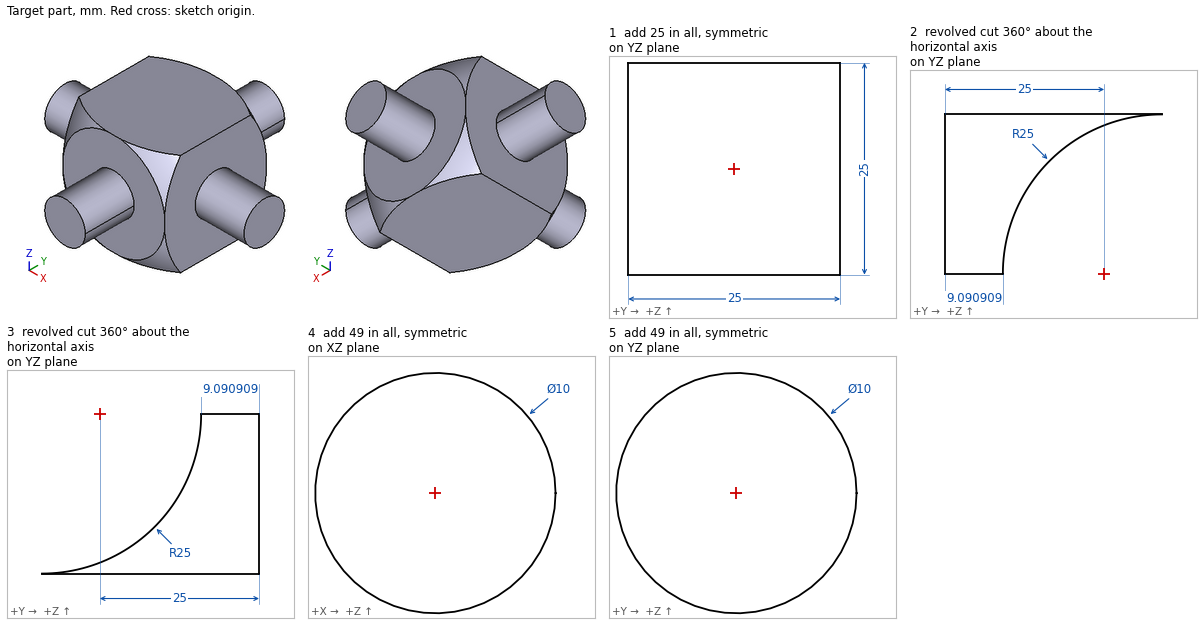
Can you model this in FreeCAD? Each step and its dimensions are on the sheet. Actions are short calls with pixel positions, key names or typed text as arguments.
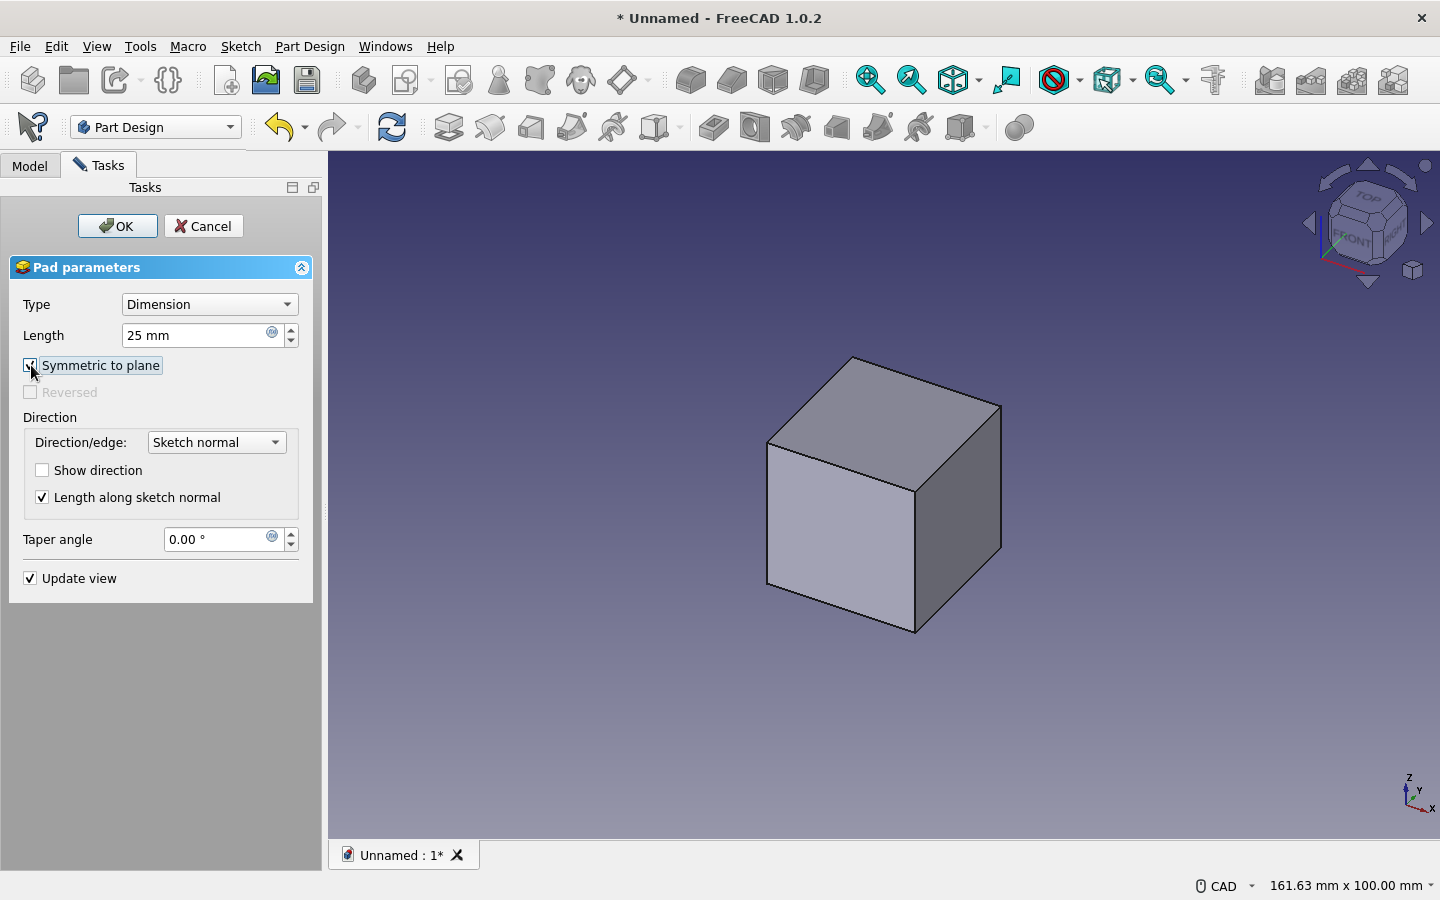
click(118, 226)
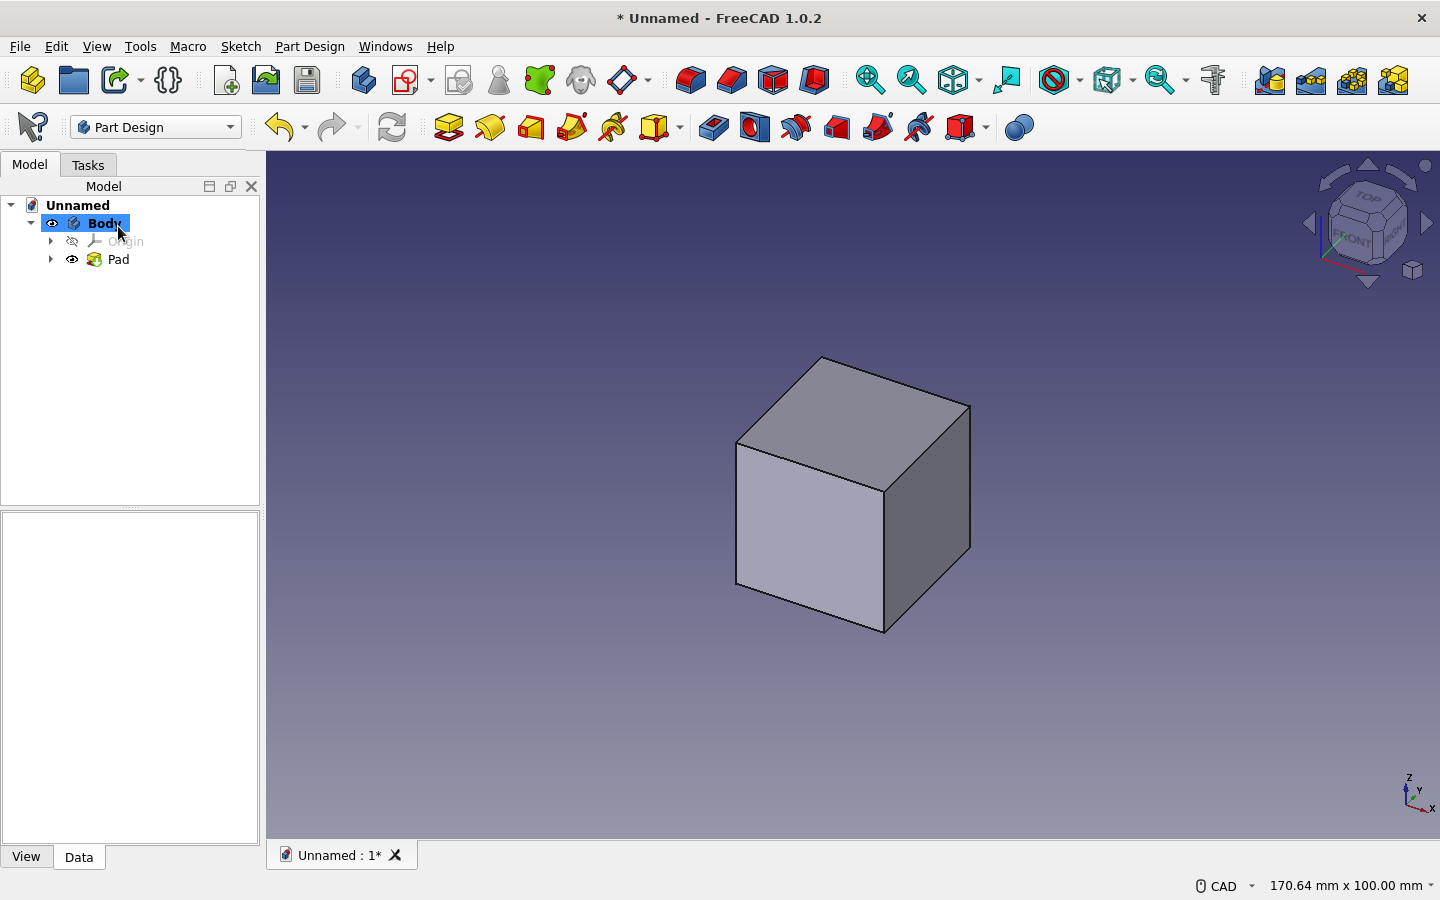
key(v)
key(f)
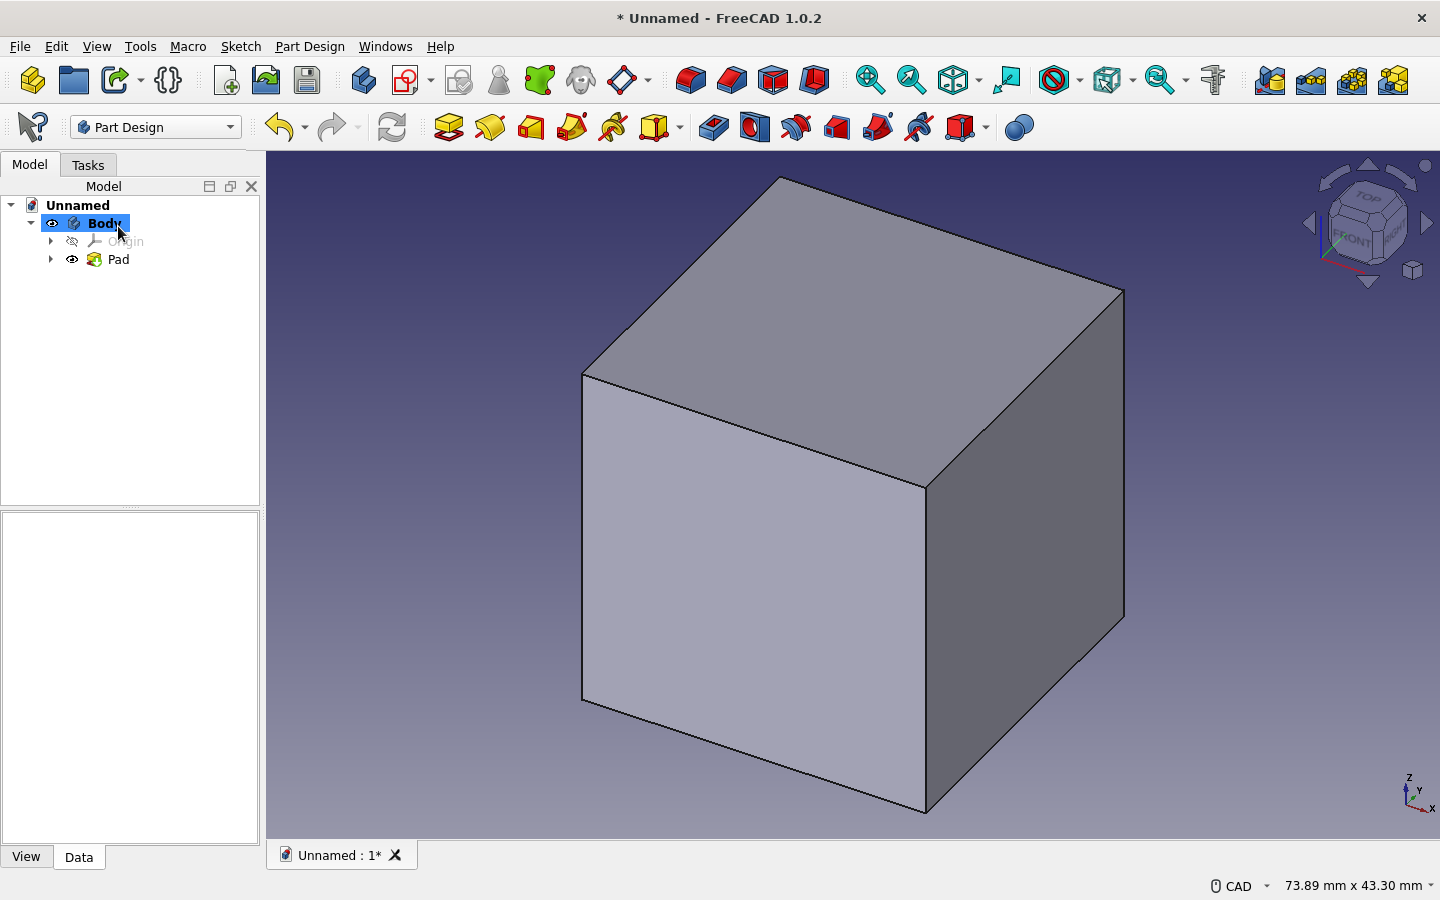
click(404, 80)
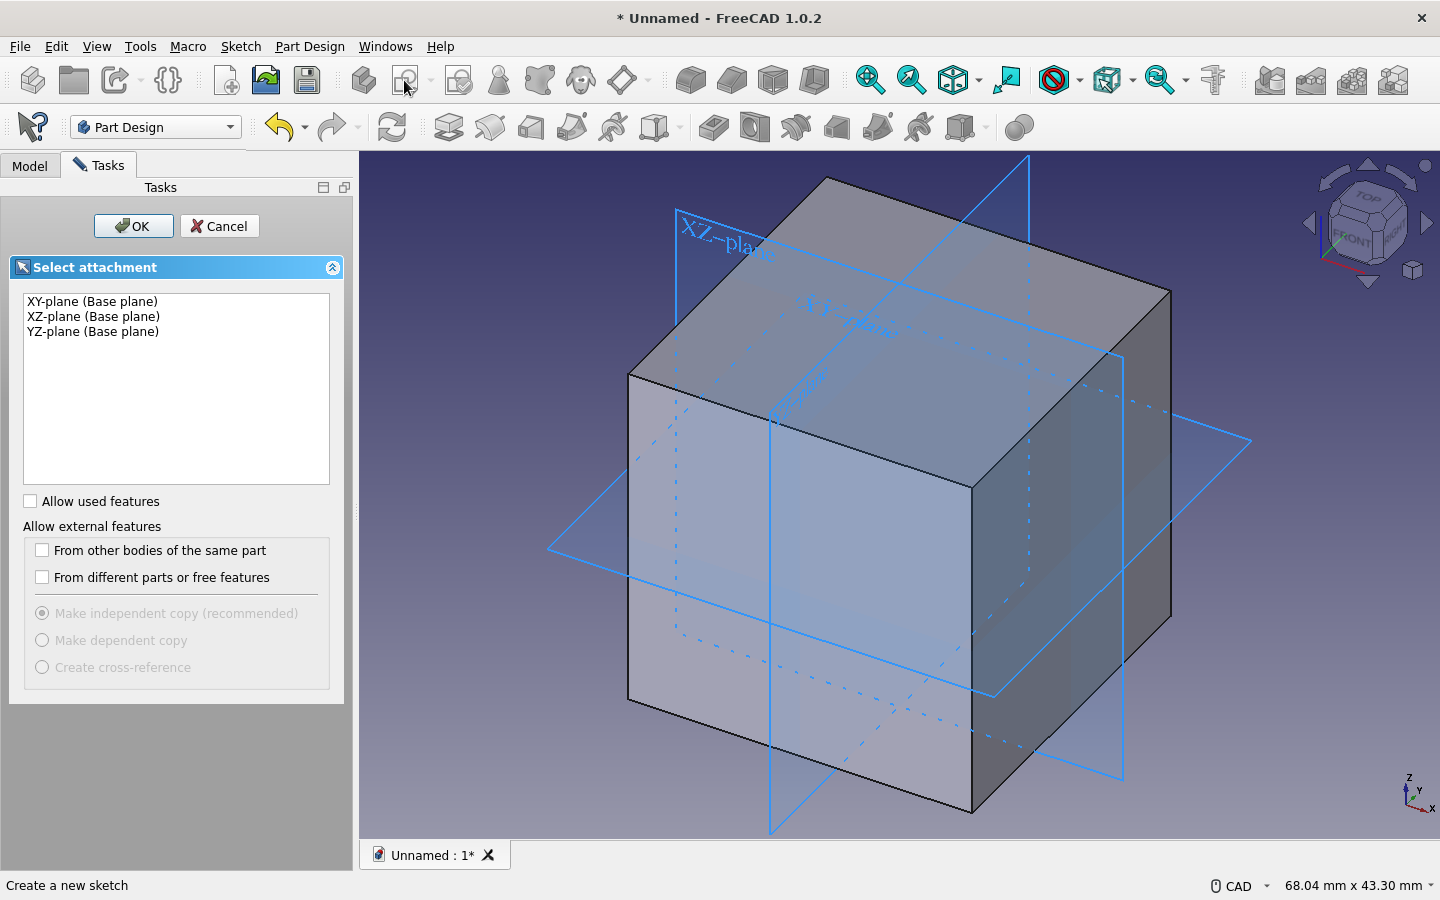
click(84, 332)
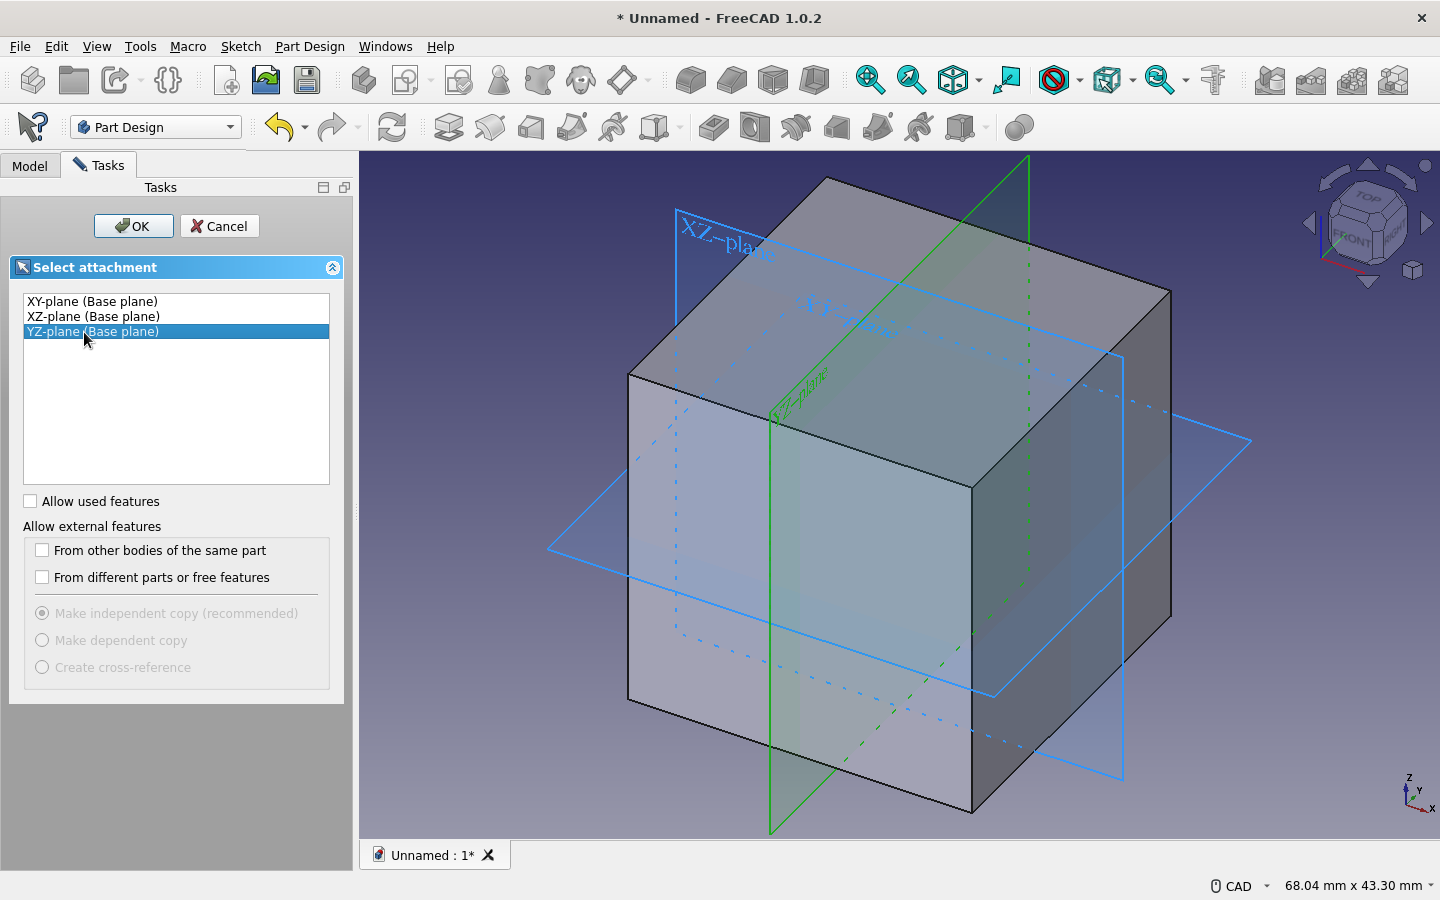
click(134, 226)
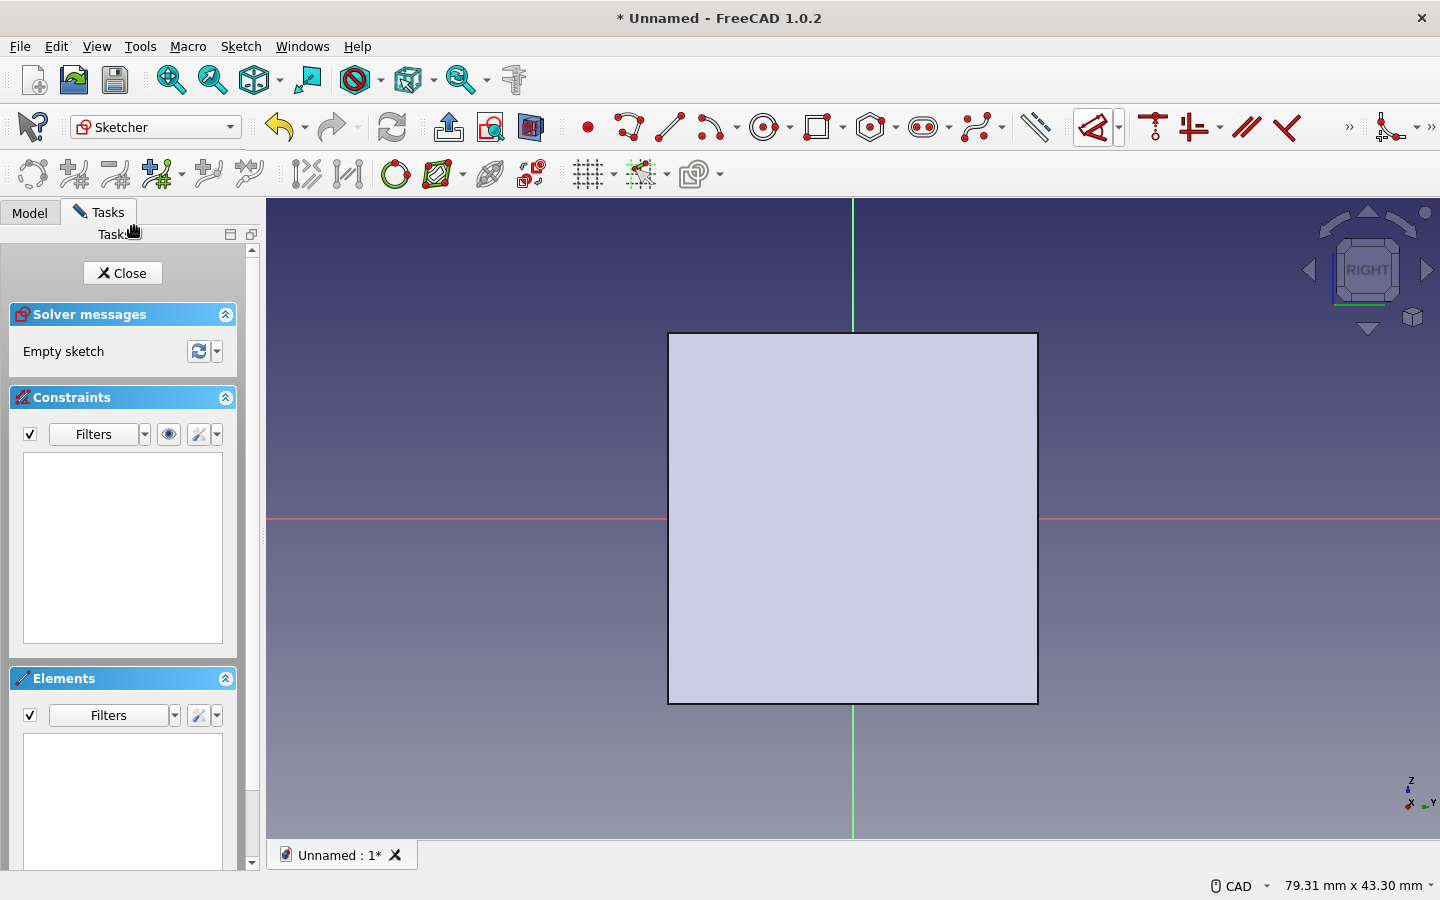
key(q)
key(s)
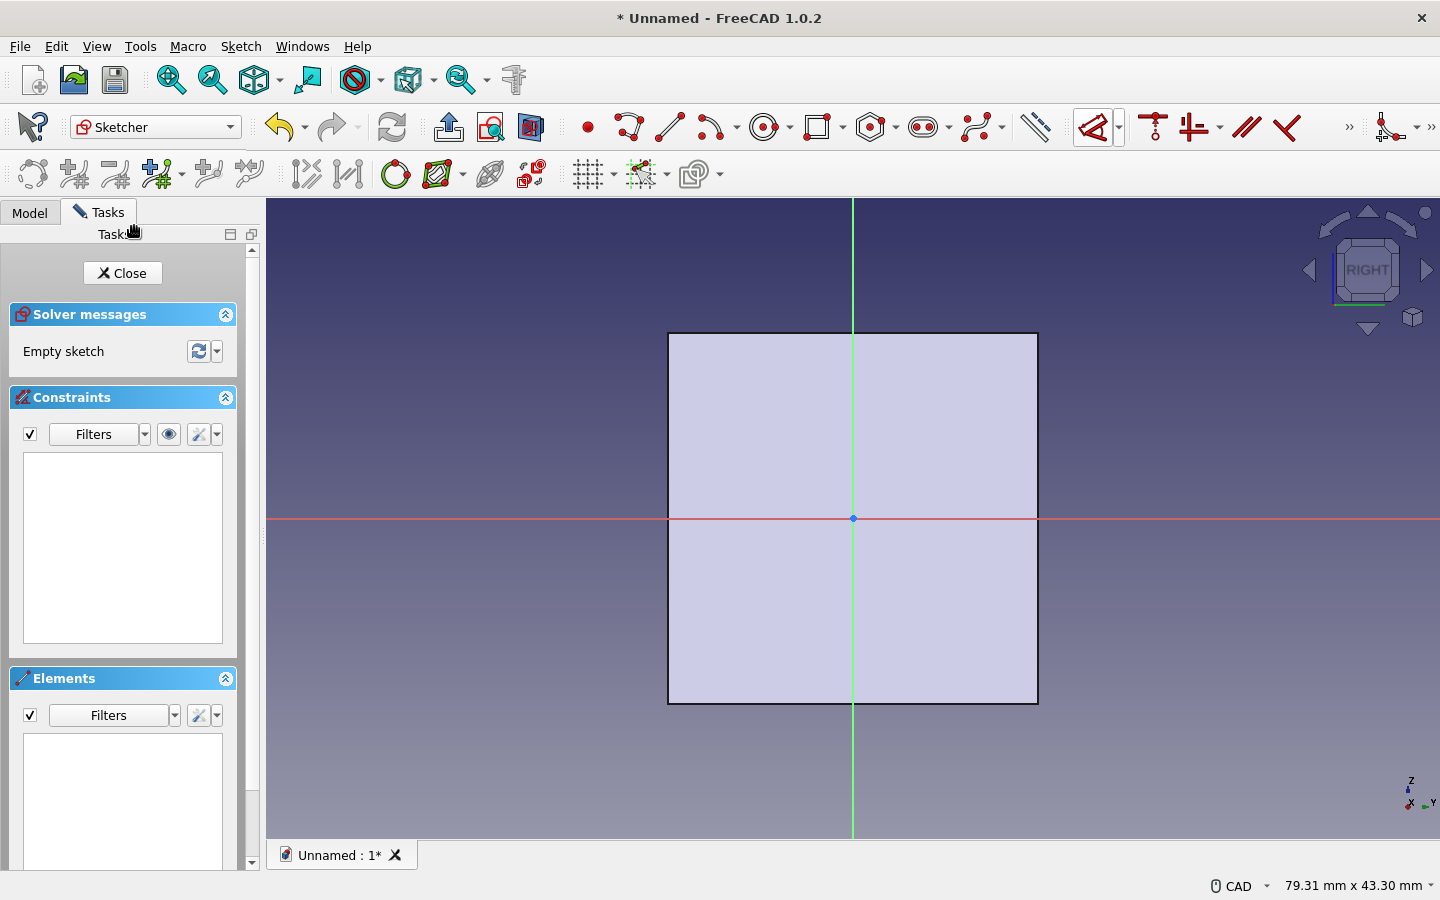
scroll(1007, 811, down, 1)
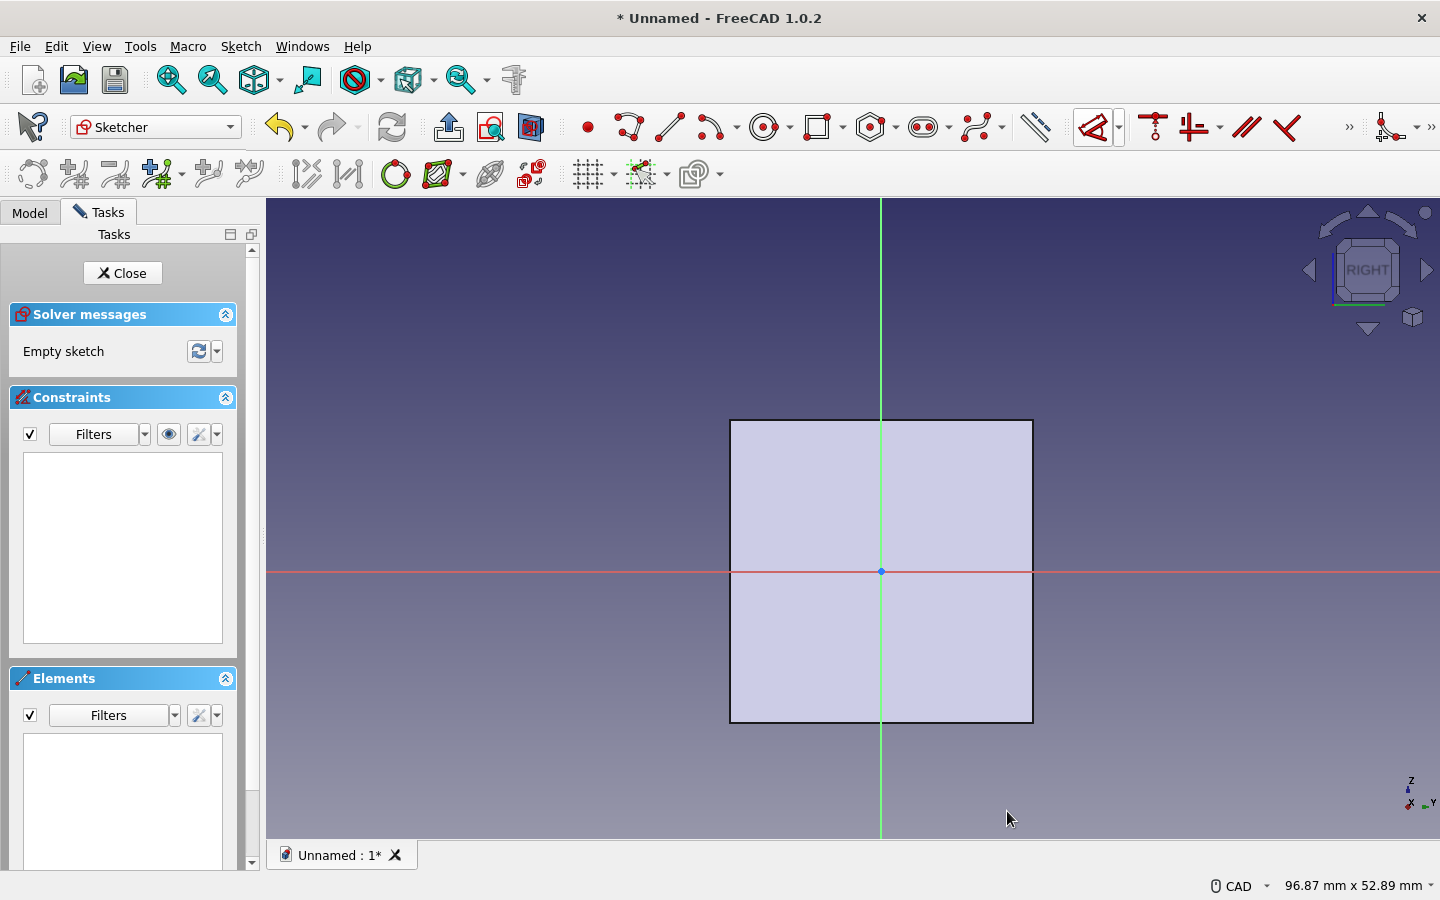
scroll(785, 226, up, 2)